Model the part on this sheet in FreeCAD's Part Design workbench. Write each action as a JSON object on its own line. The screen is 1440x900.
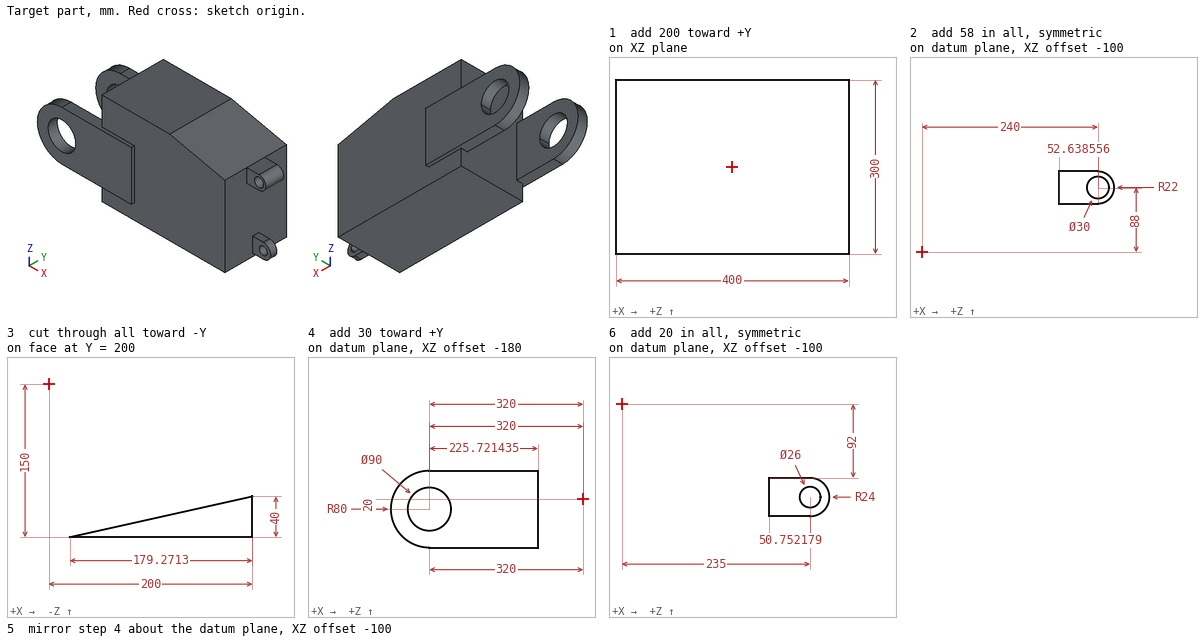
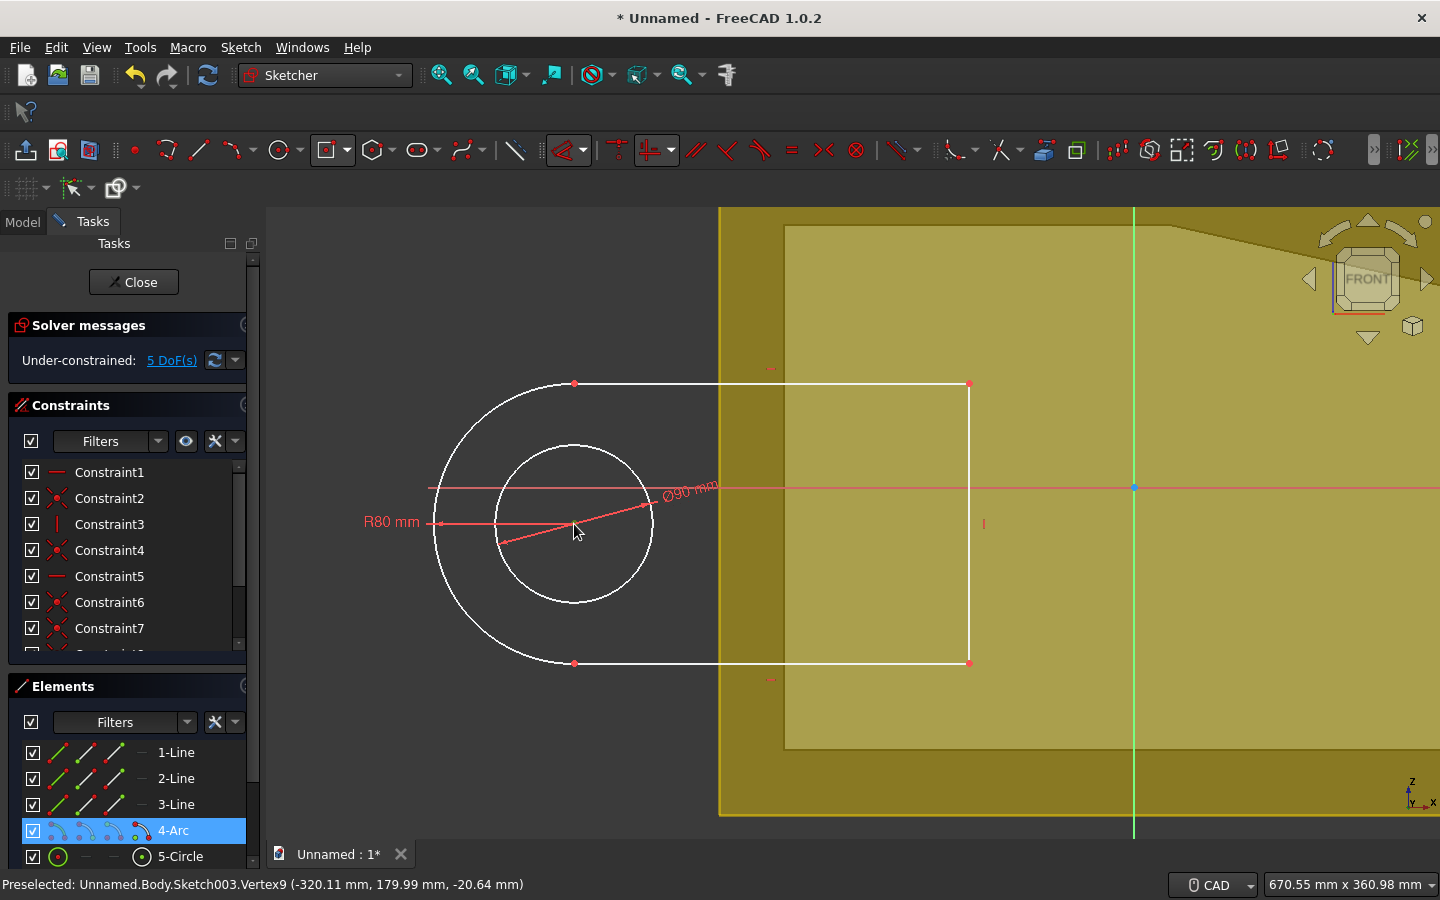
{"action": "key", "text": "i"}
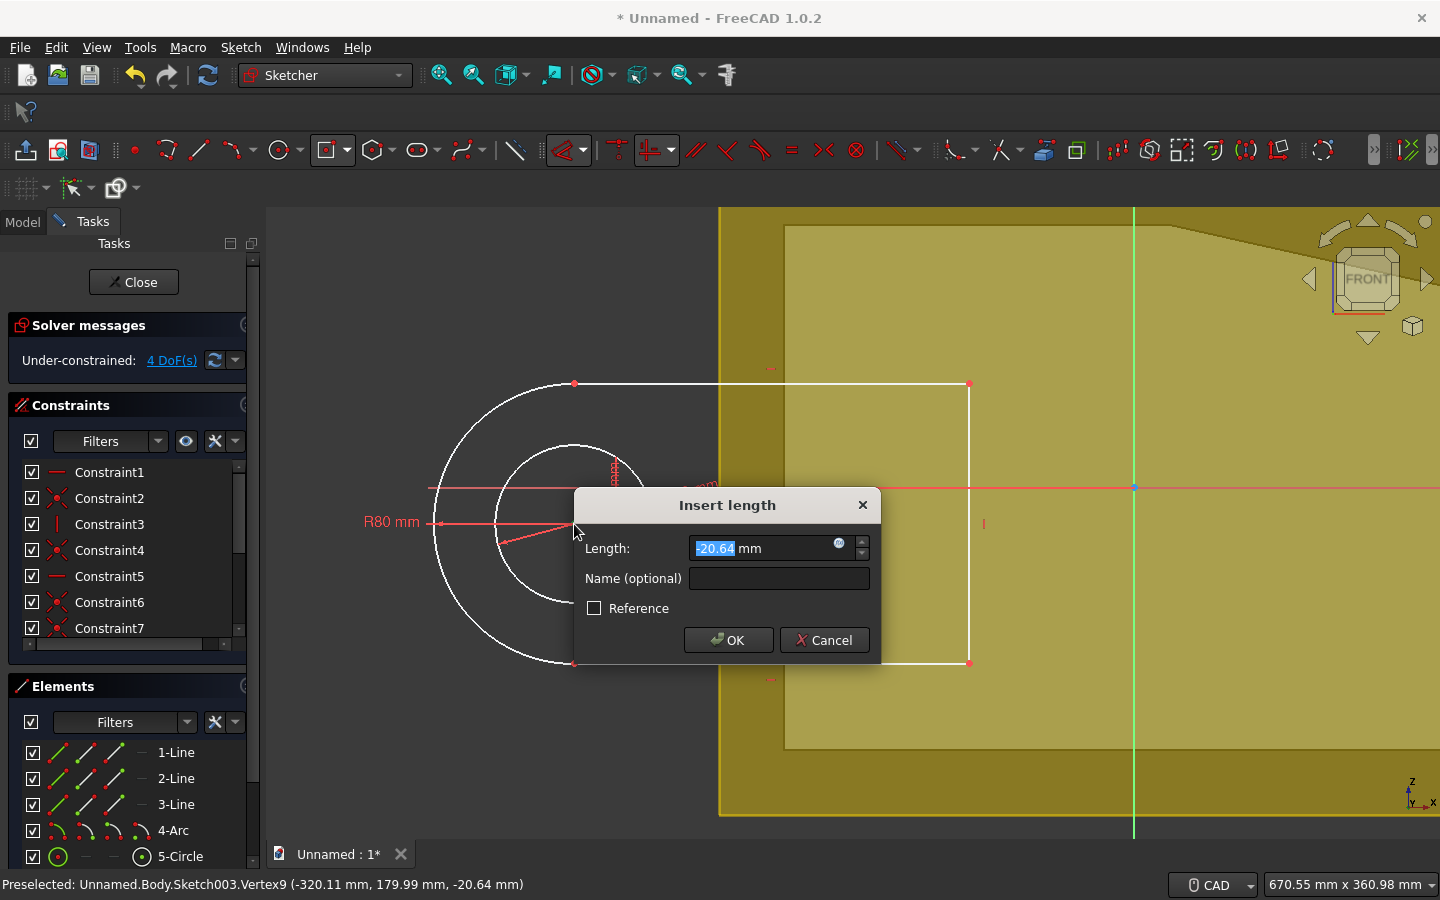
{"action": "type", "text": "-20"}
{"action": "key", "text": "Return"}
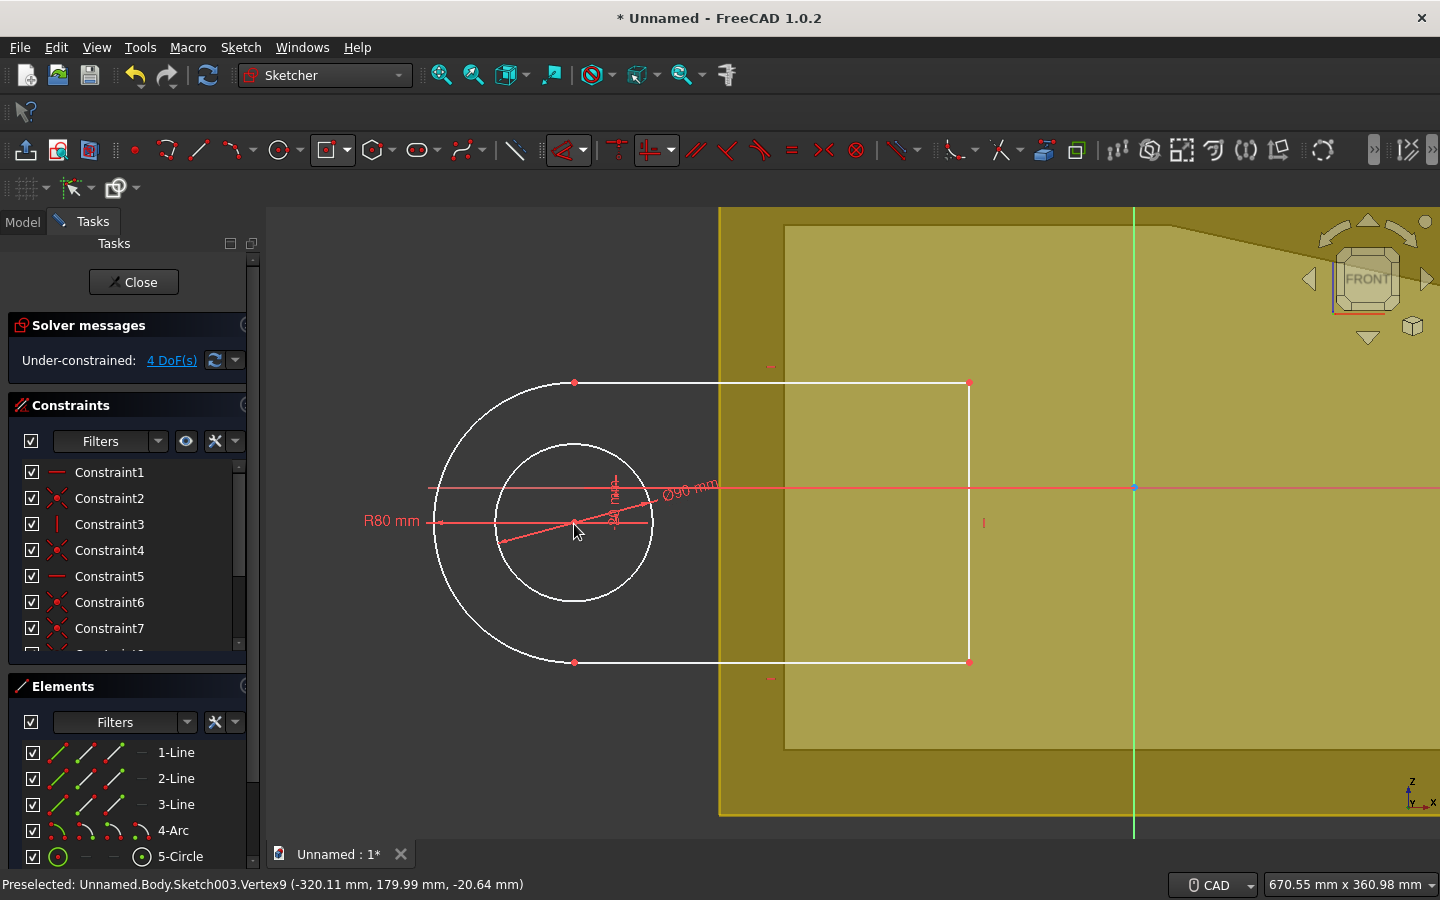
{"action": "left_click", "coordinate": [574, 523]}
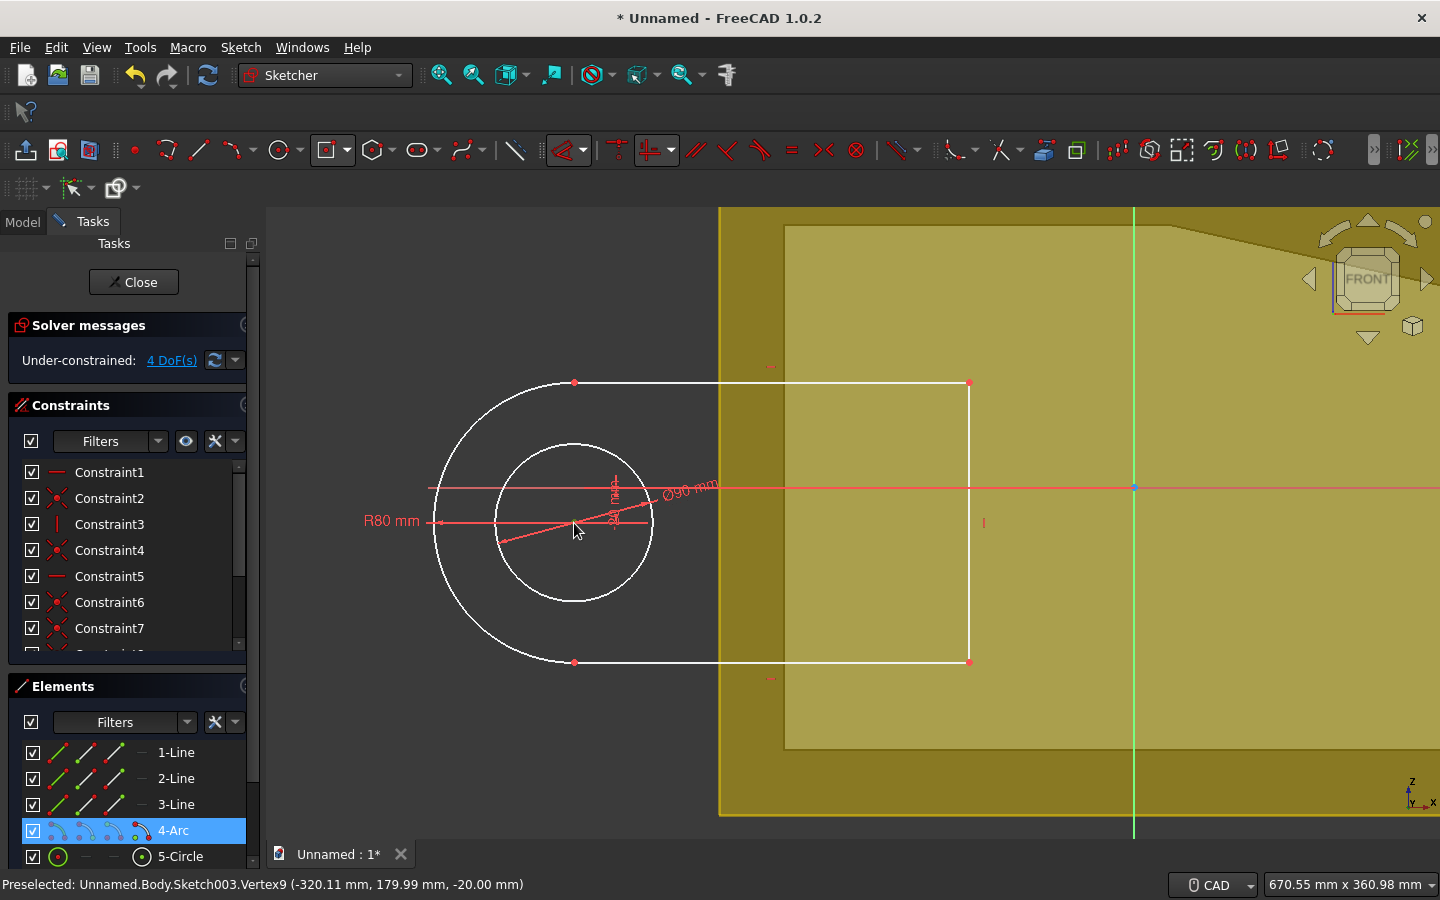
{"action": "left_click", "coordinate": [586, 150]}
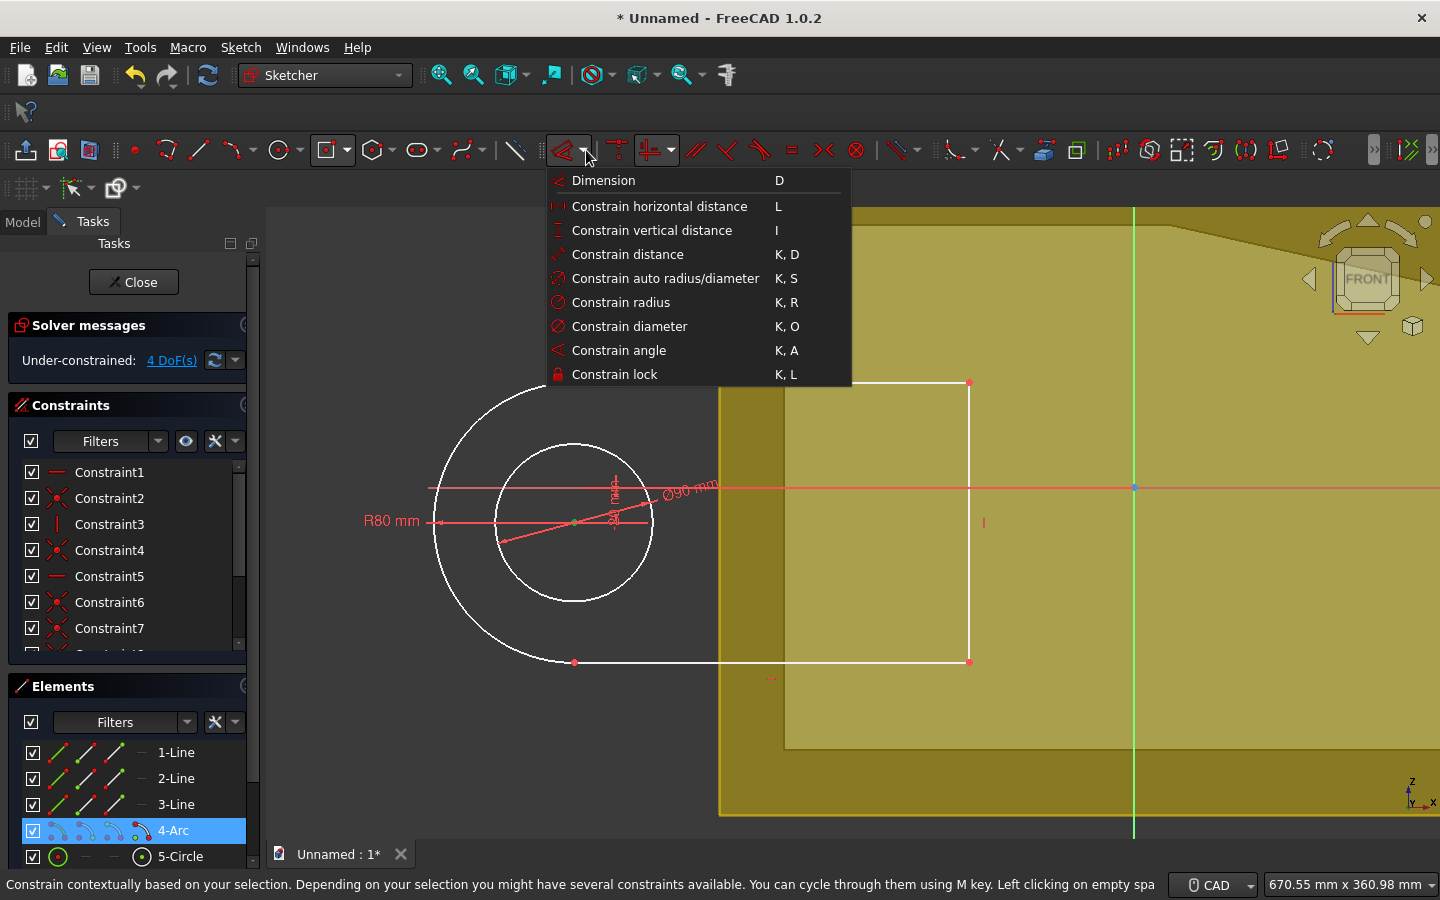
{"action": "left_click", "coordinate": [699, 206]}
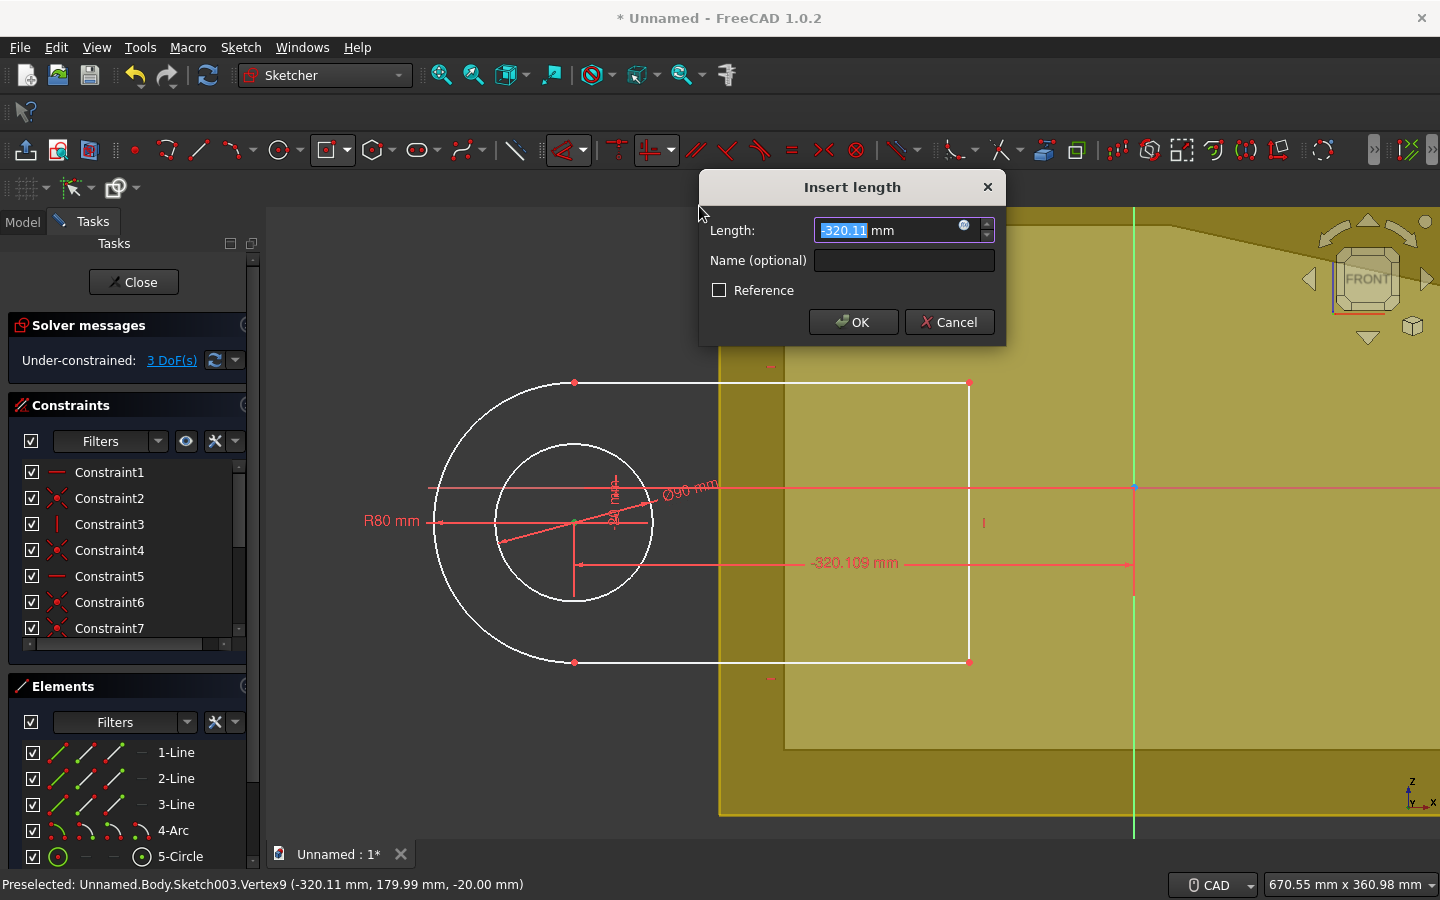
{"action": "type", "text": "-320"}
{"action": "key", "text": "Return"}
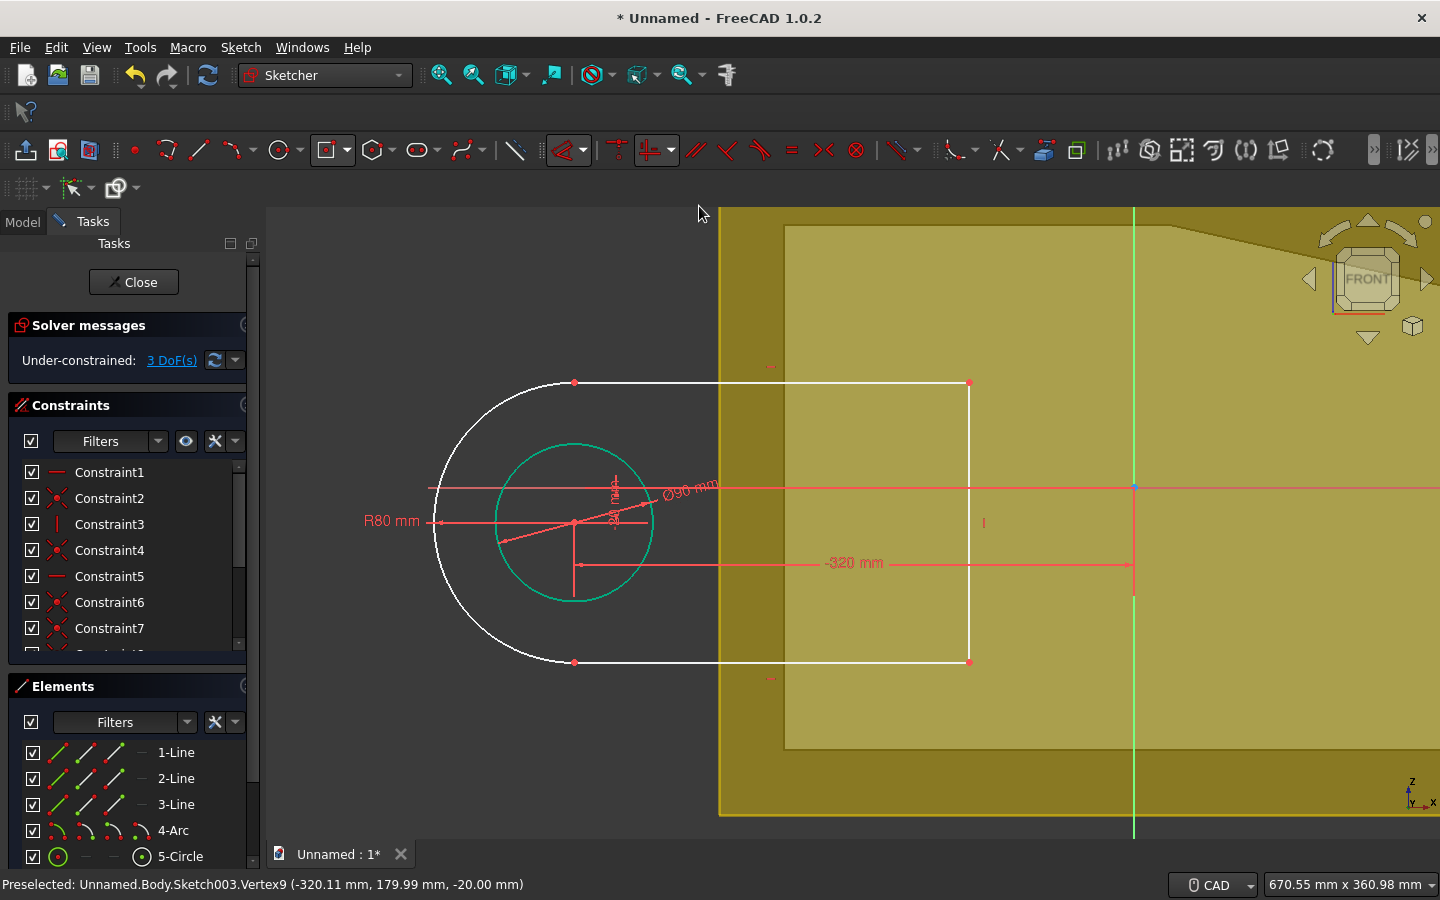
{"action": "left_click", "coordinate": [574, 383]}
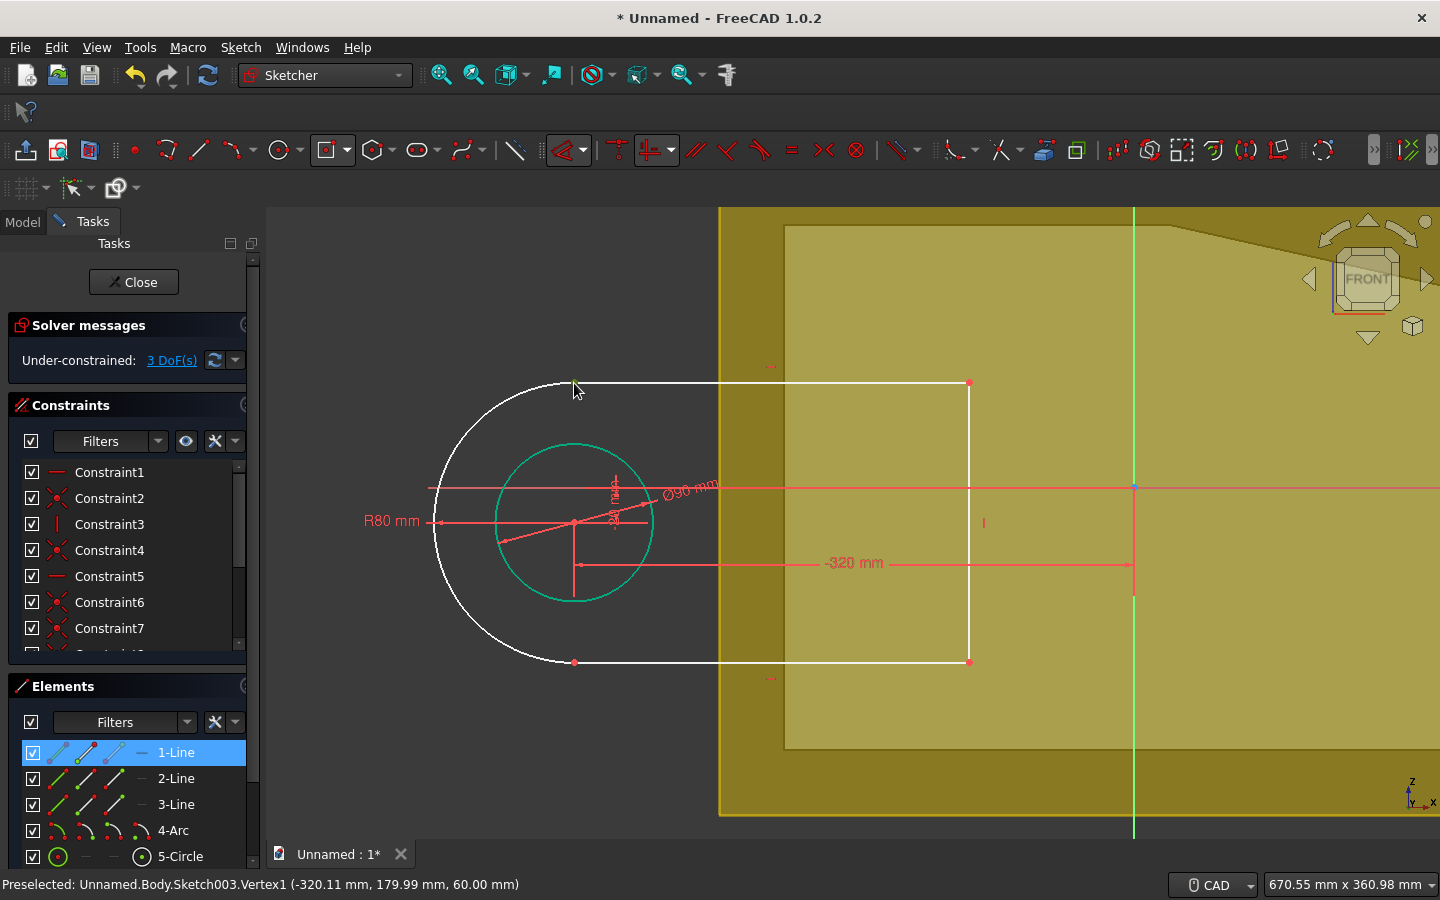
{"action": "left_click", "coordinate": [586, 150]}